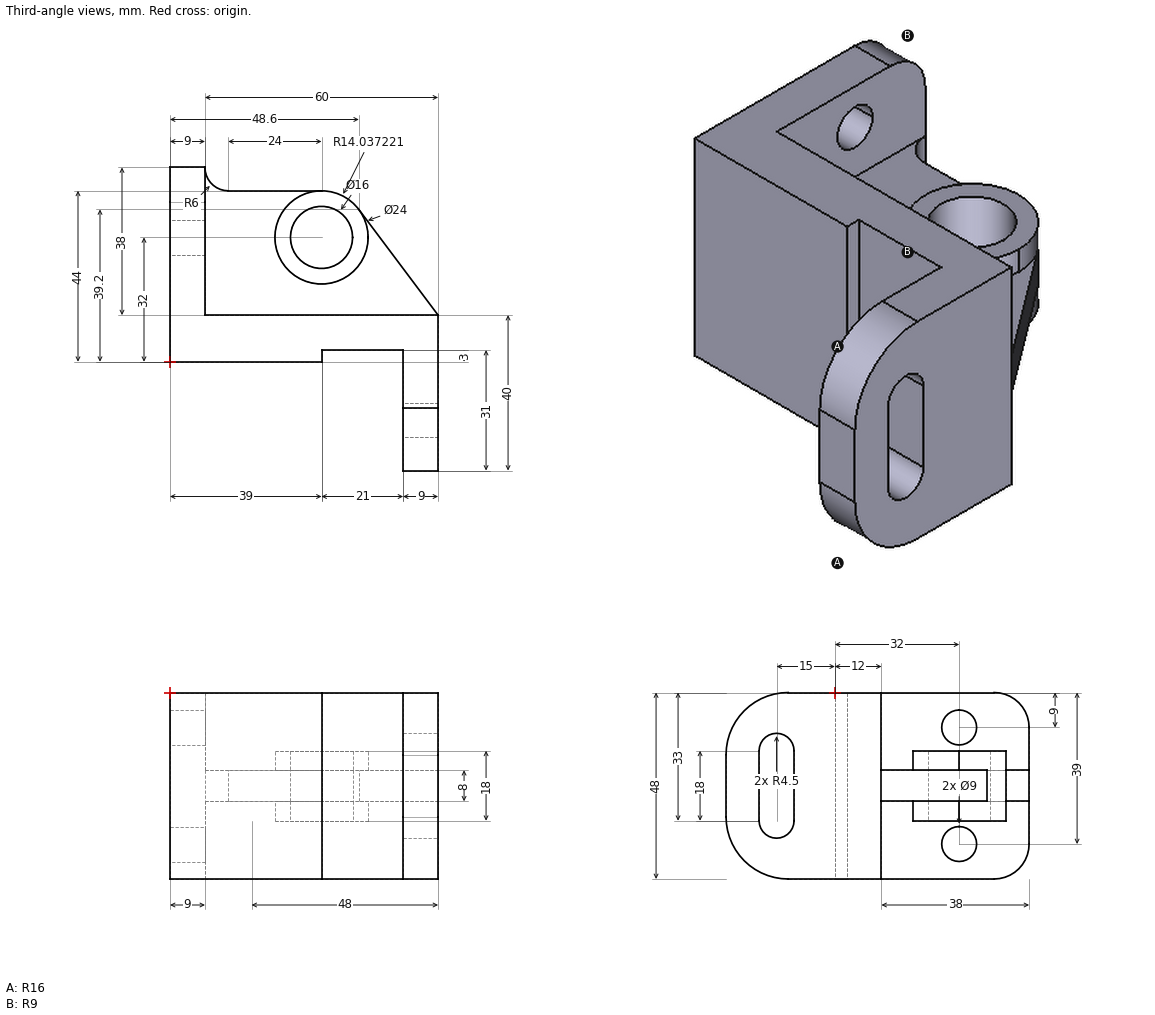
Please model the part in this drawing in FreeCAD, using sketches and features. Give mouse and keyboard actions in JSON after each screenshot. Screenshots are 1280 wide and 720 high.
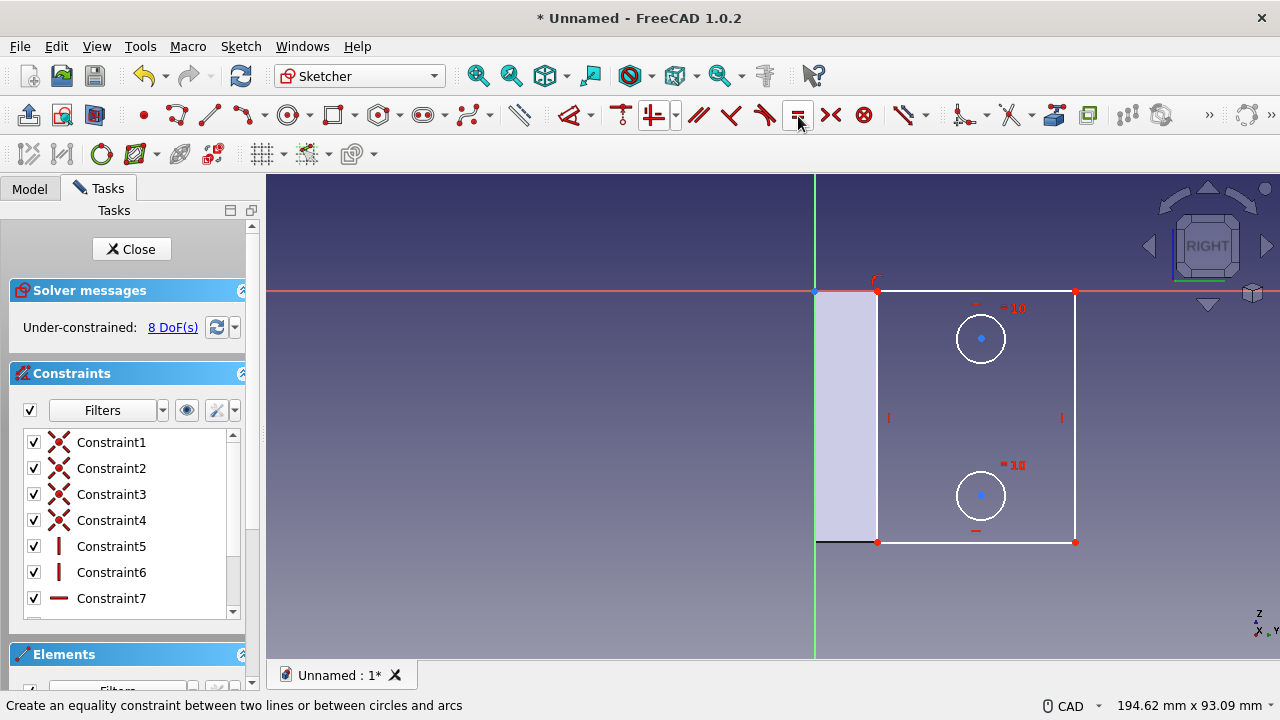
{"action": "left_click", "coordinate": [981, 496]}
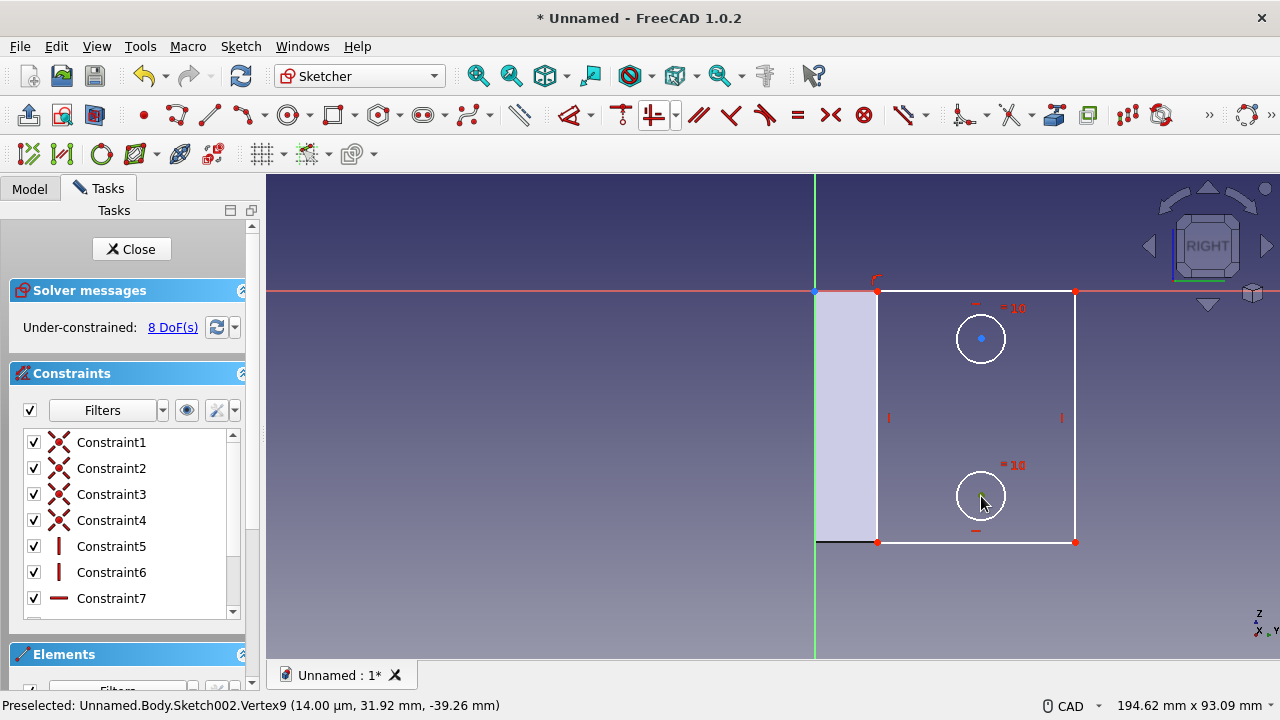
{"action": "left_click", "coordinate": [981, 339]}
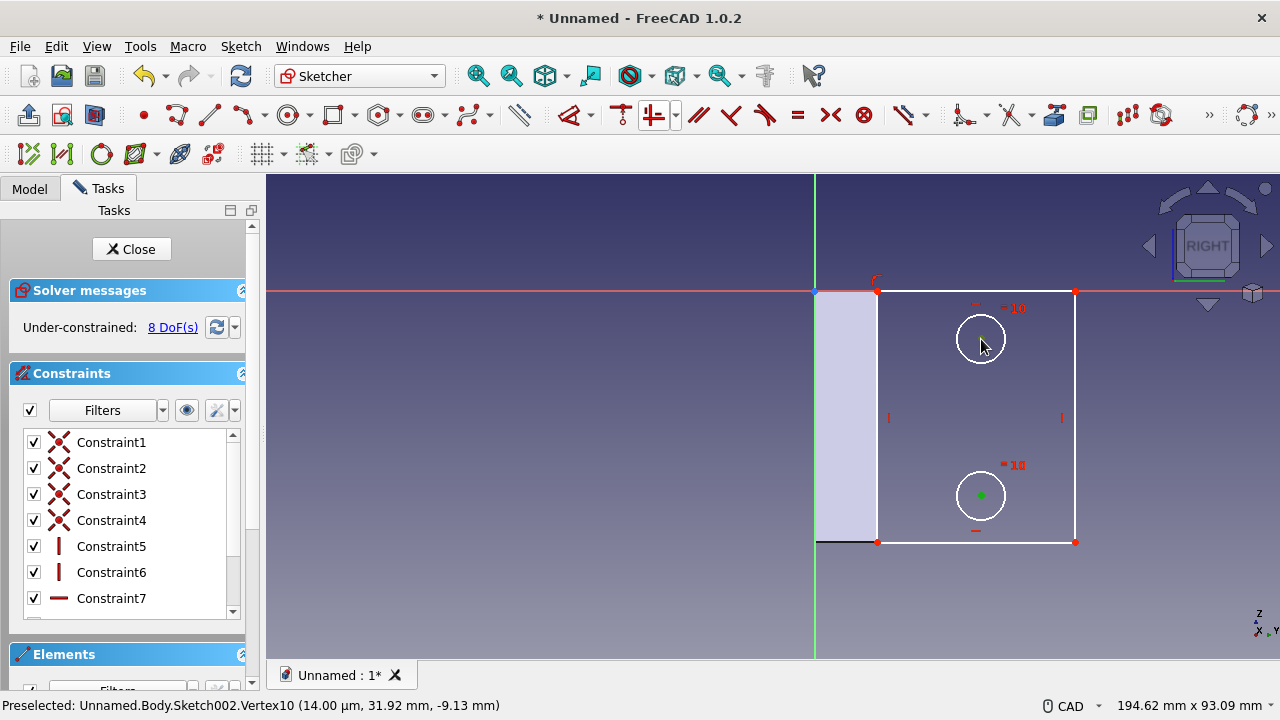
{"action": "key", "text": "v"}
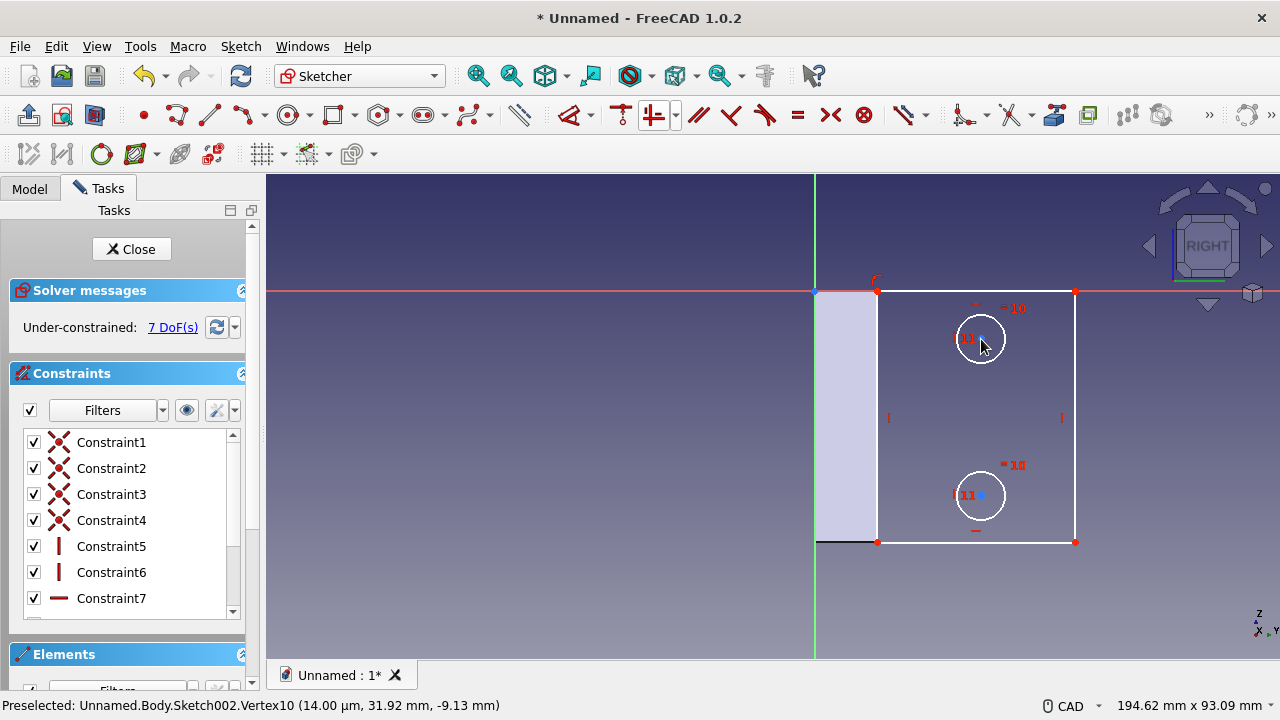
{"action": "key", "text": "d"}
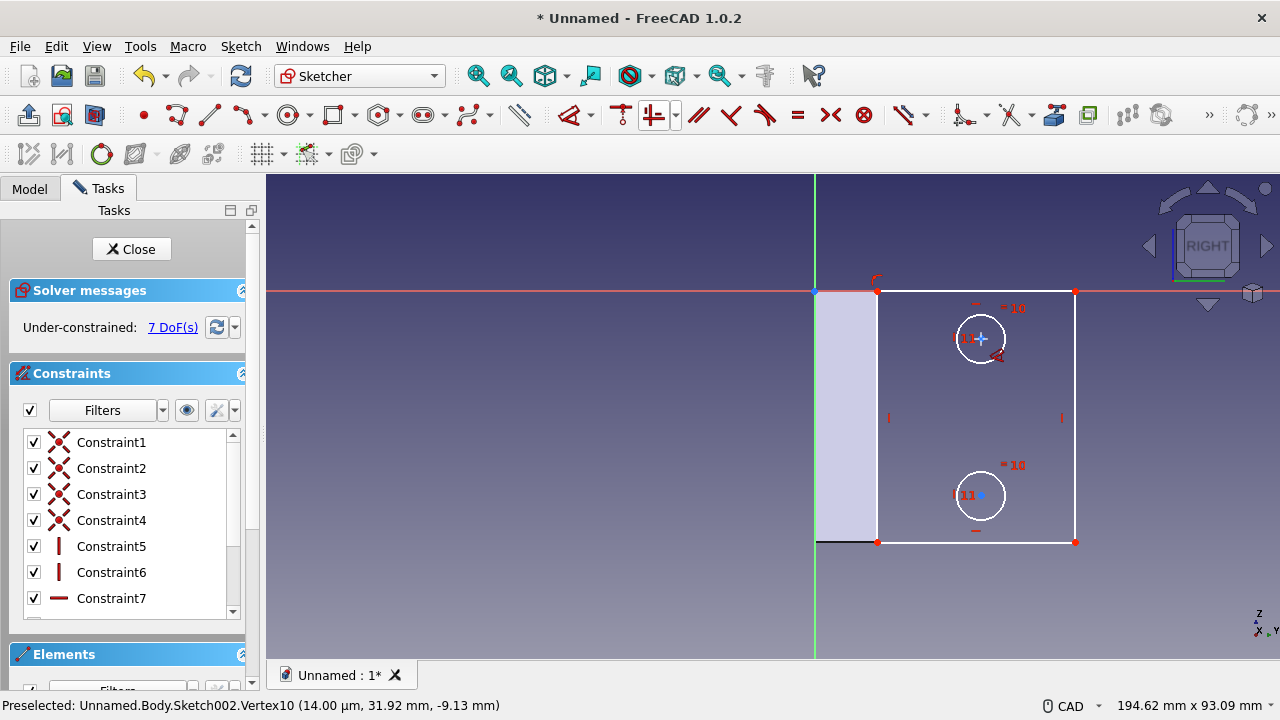
{"action": "left_click", "coordinate": [998, 479]}
{"action": "left_click", "coordinate": [1021, 456]}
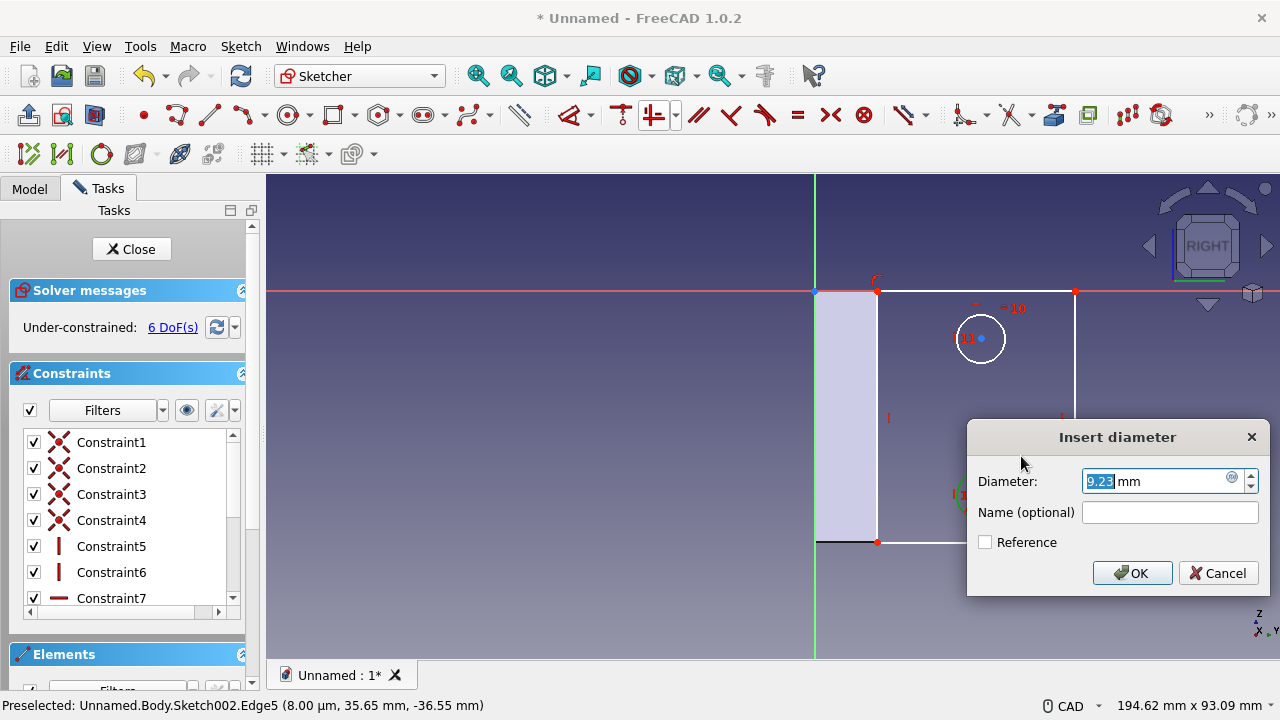
{"action": "type", "text": "9"}
{"action": "key", "text": "Return"}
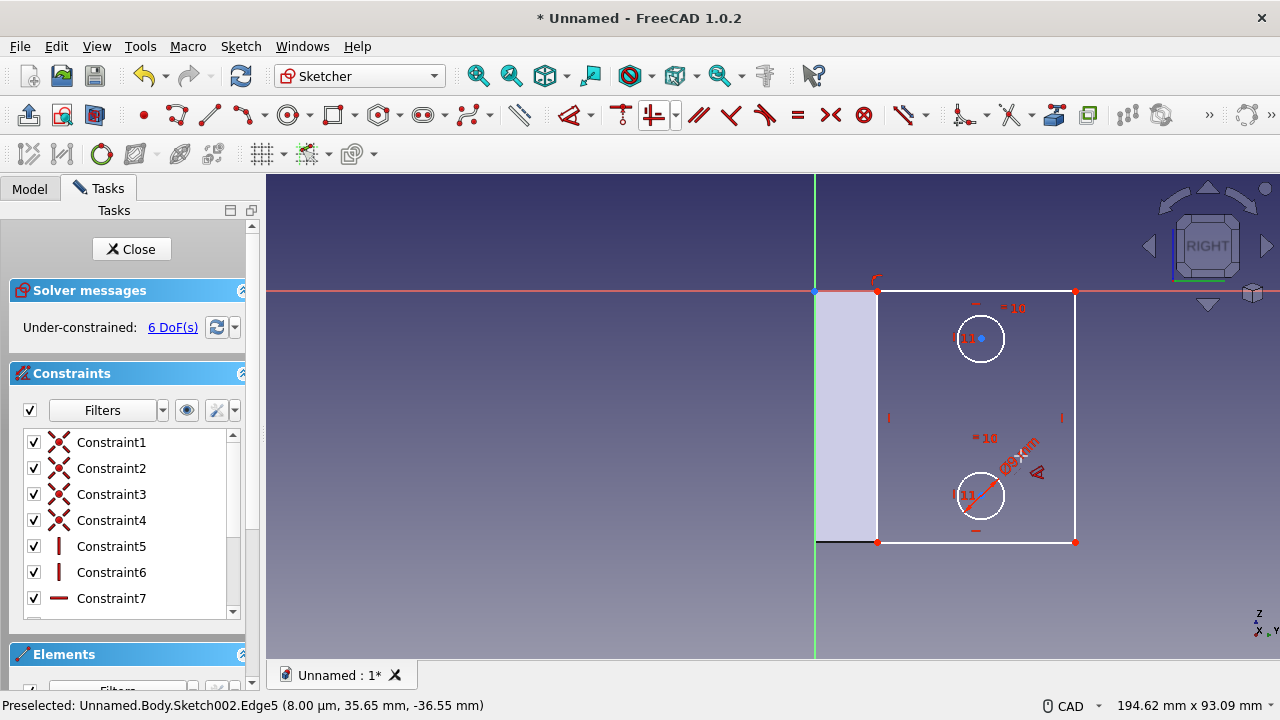
{"action": "left_click", "coordinate": [981, 339]}
{"action": "left_click", "coordinate": [781, 315]}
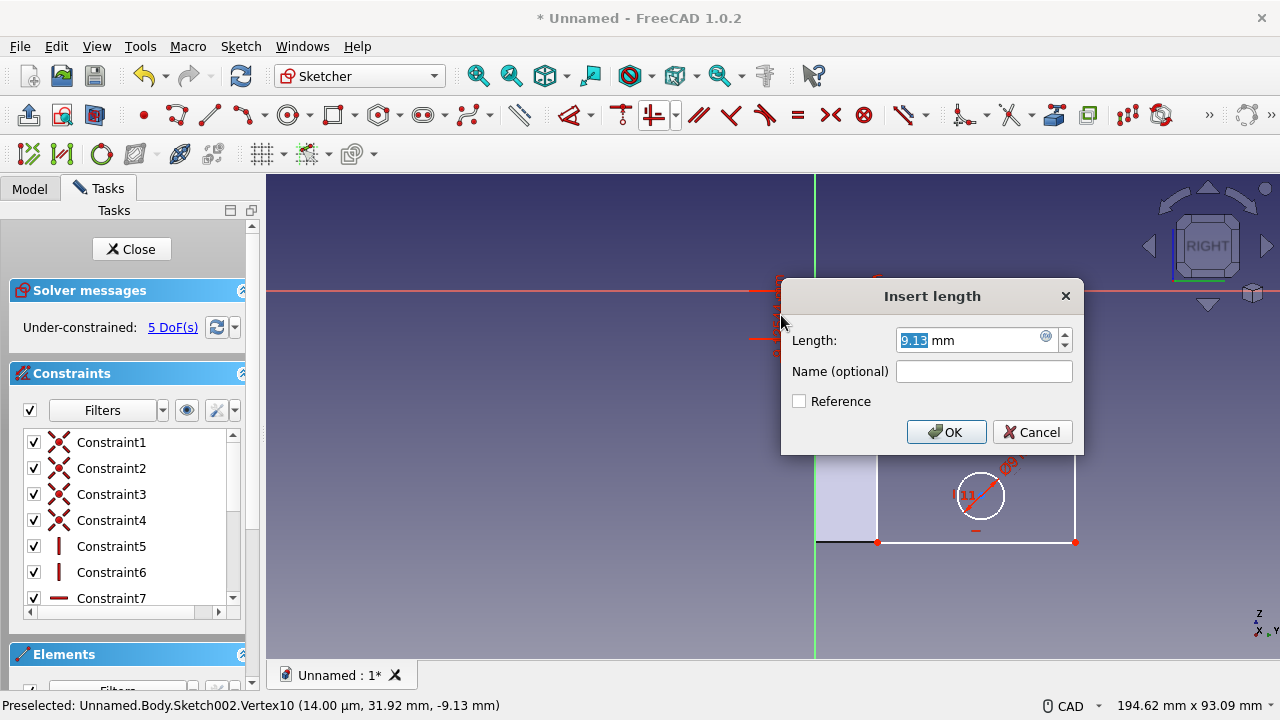
{"action": "type", "text": "9"}
{"action": "key", "text": "Return"}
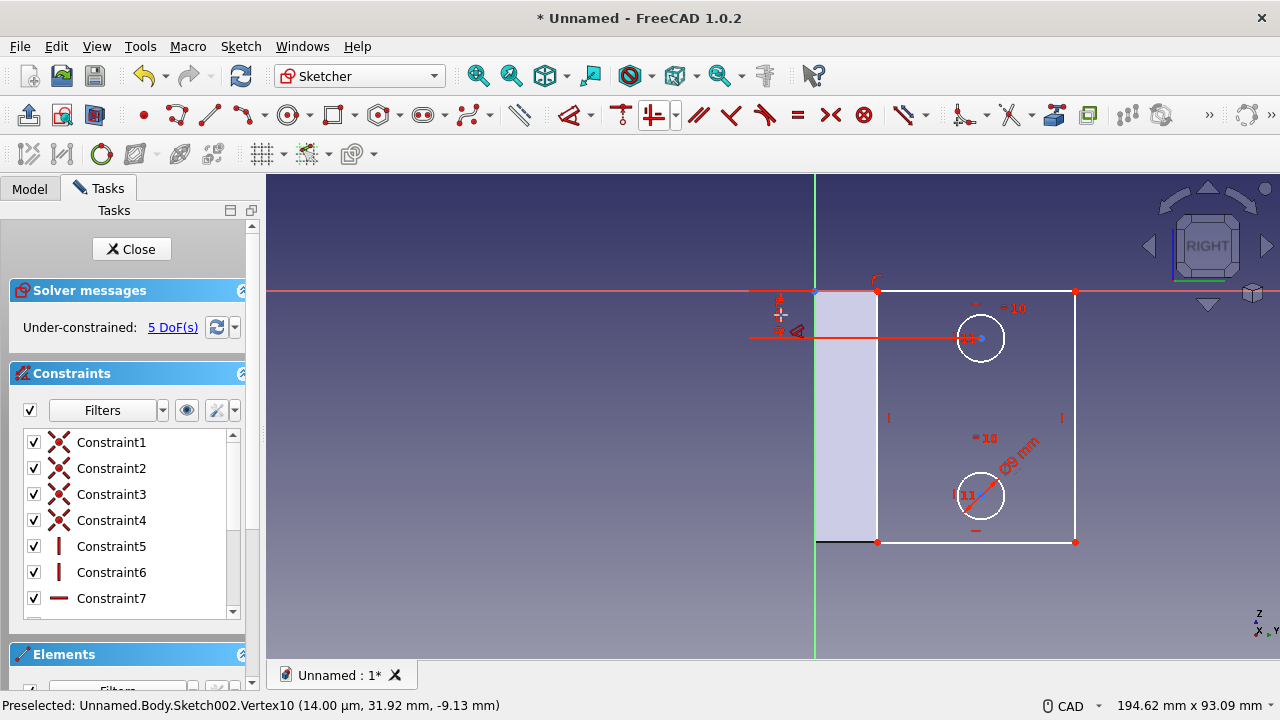
{"action": "left_click", "coordinate": [877, 367]}
{"action": "left_click", "coordinate": [843, 417]}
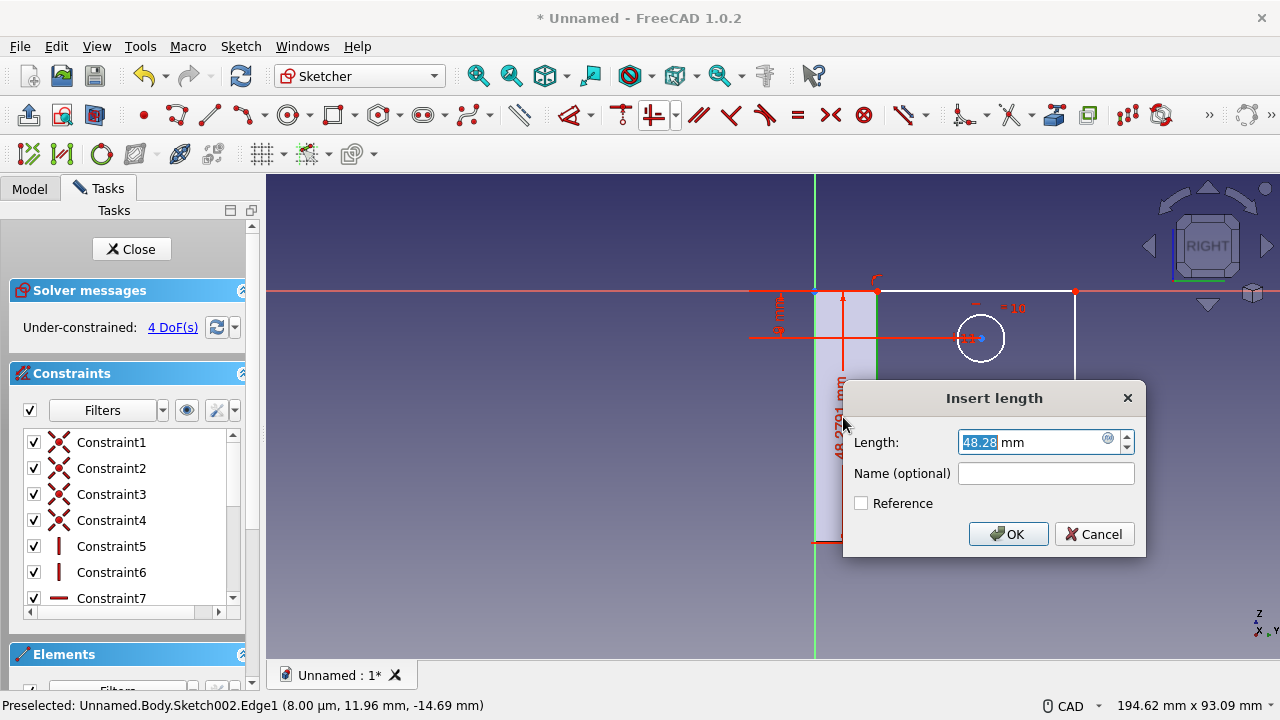
{"action": "type", "text": "48"}
{"action": "key", "text": "Return"}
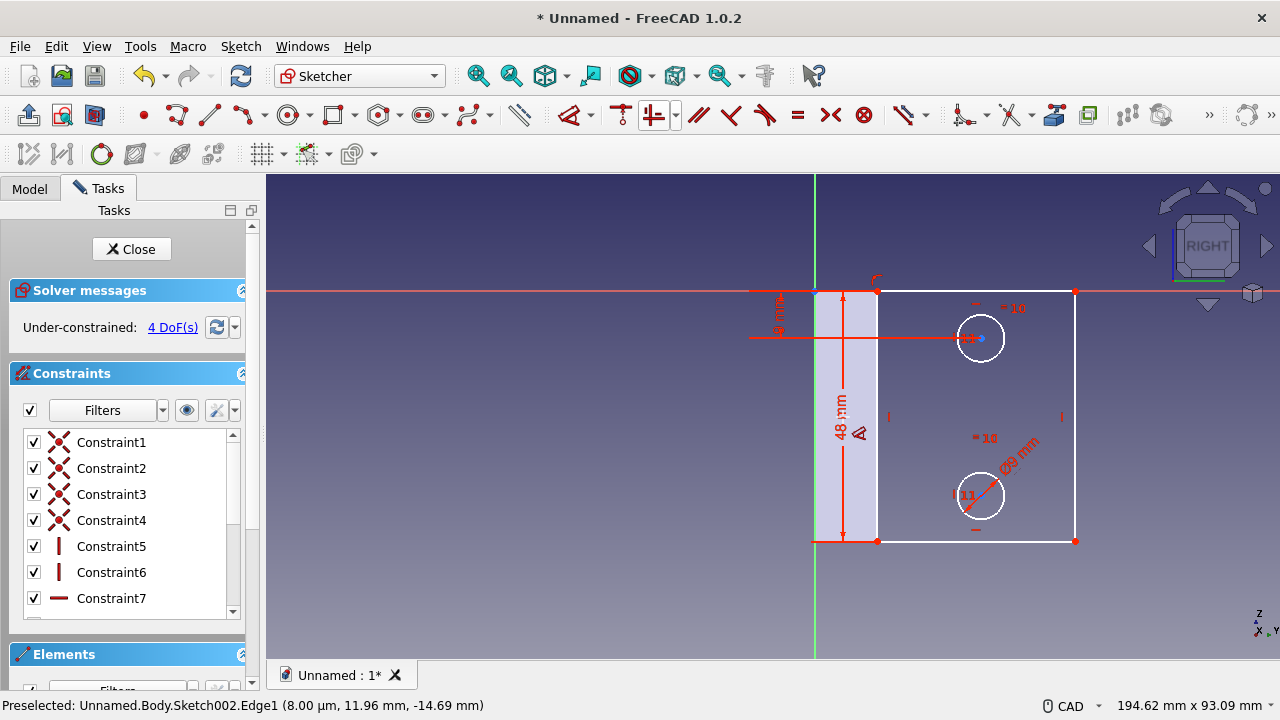
{"action": "left_click", "coordinate": [936, 542]}
{"action": "left_click", "coordinate": [976, 576]}